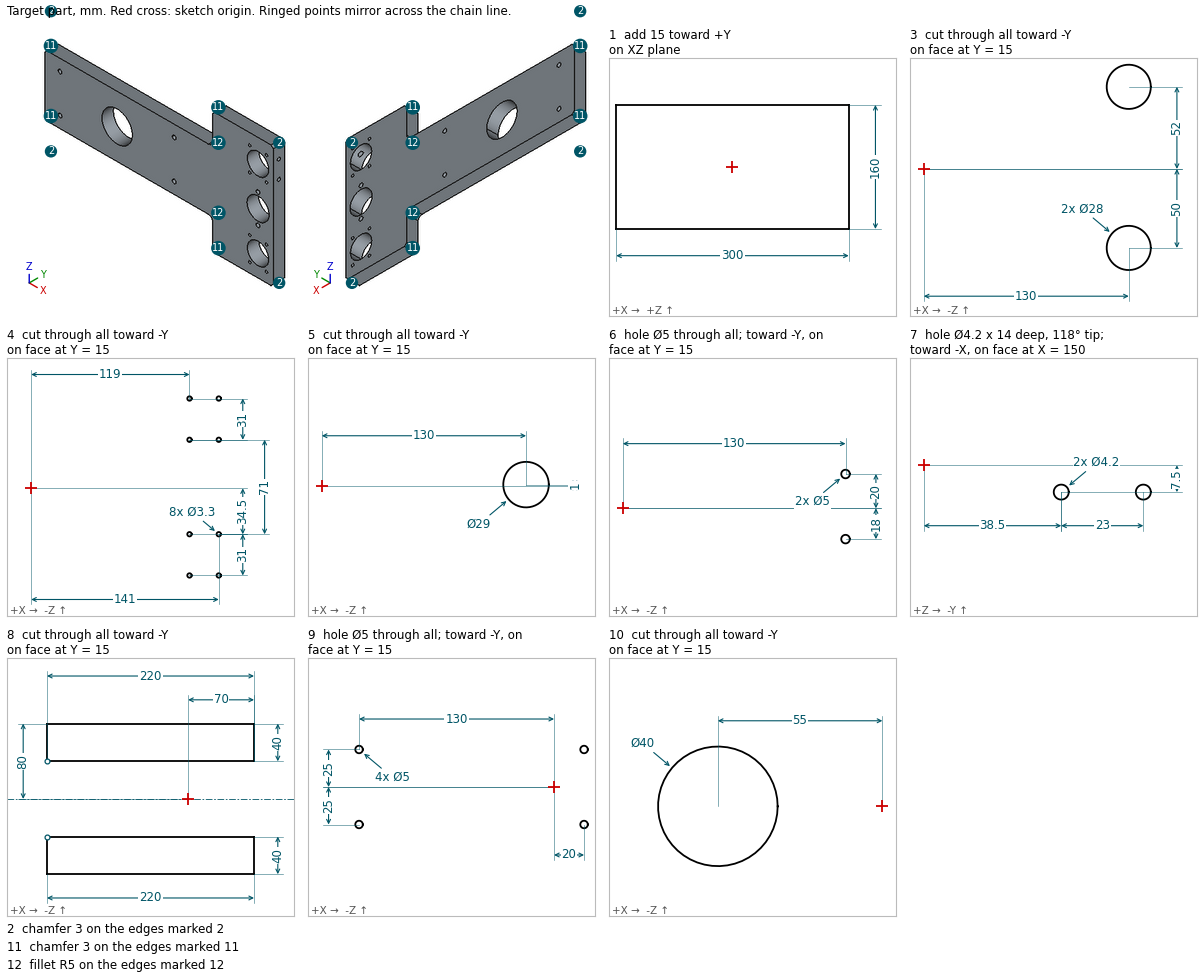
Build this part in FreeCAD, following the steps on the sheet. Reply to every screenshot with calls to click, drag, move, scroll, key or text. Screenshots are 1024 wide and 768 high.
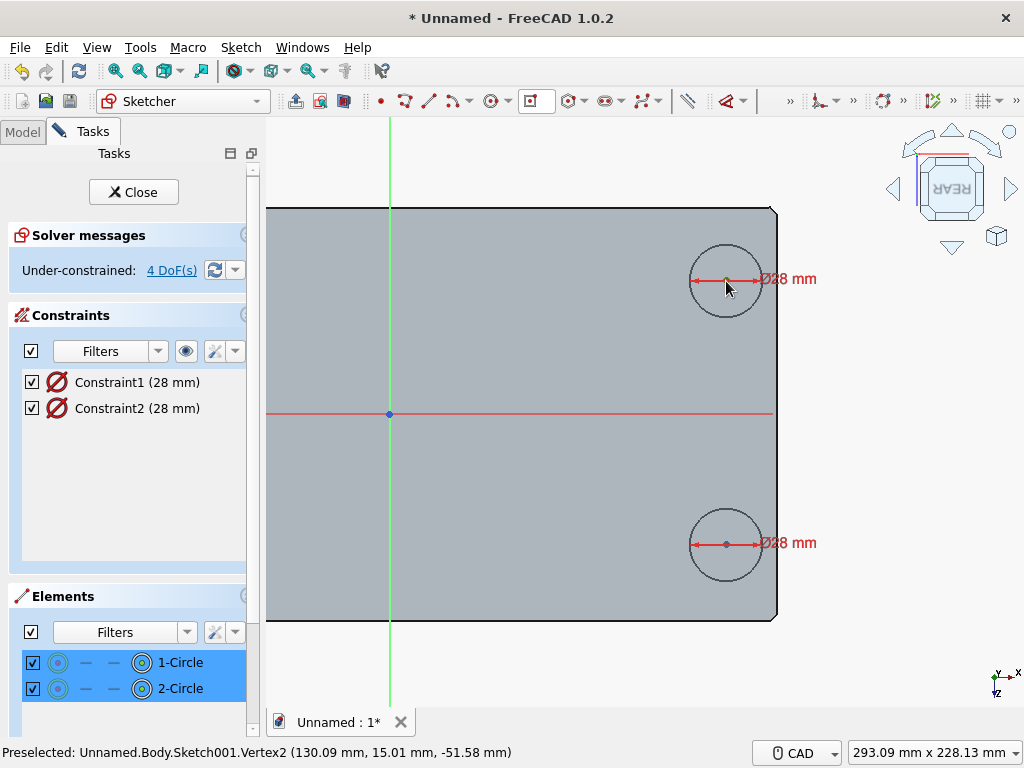
key(v)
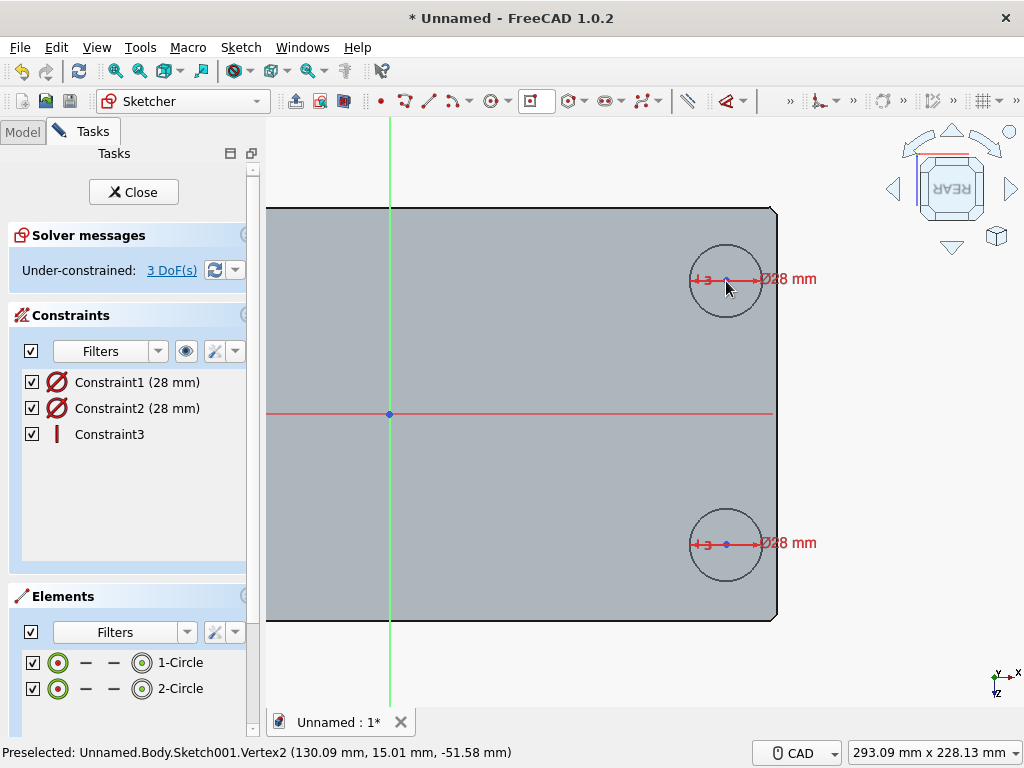
click(726, 102)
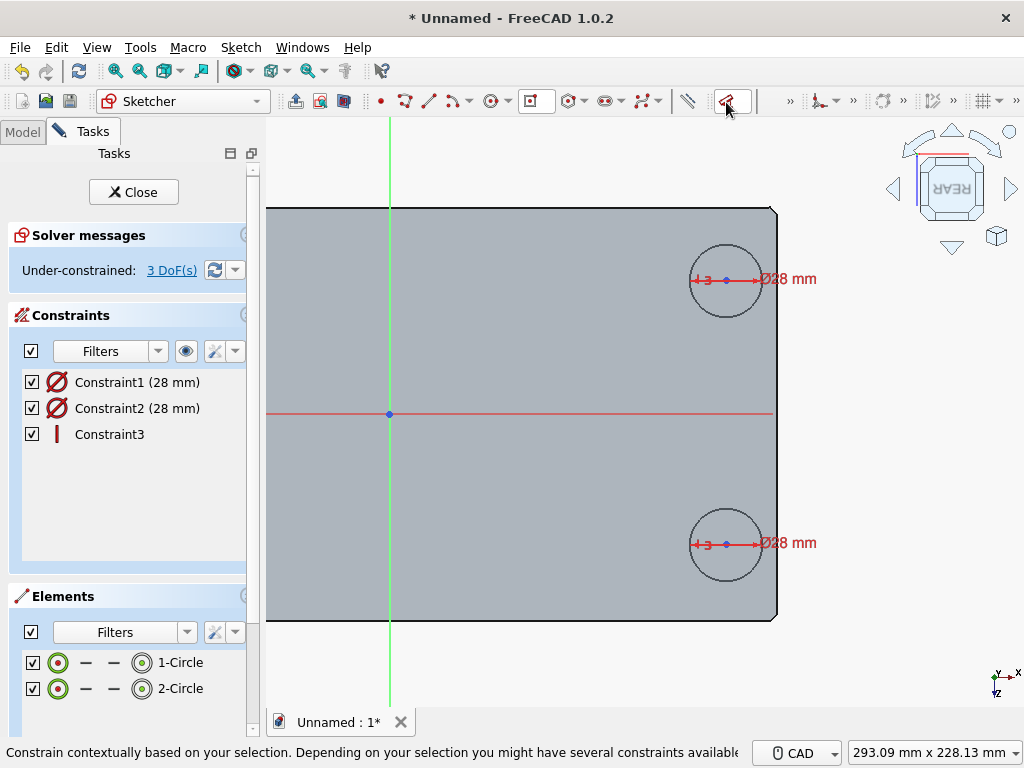
click(726, 545)
click(356, 480)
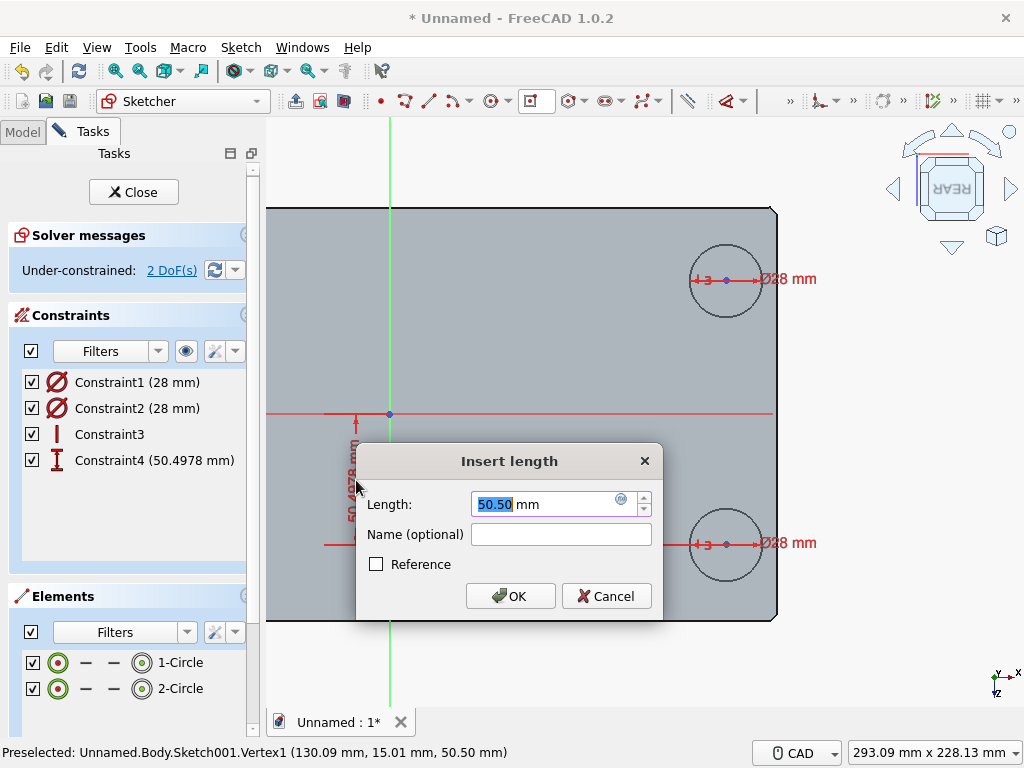
text(50)
key(Return)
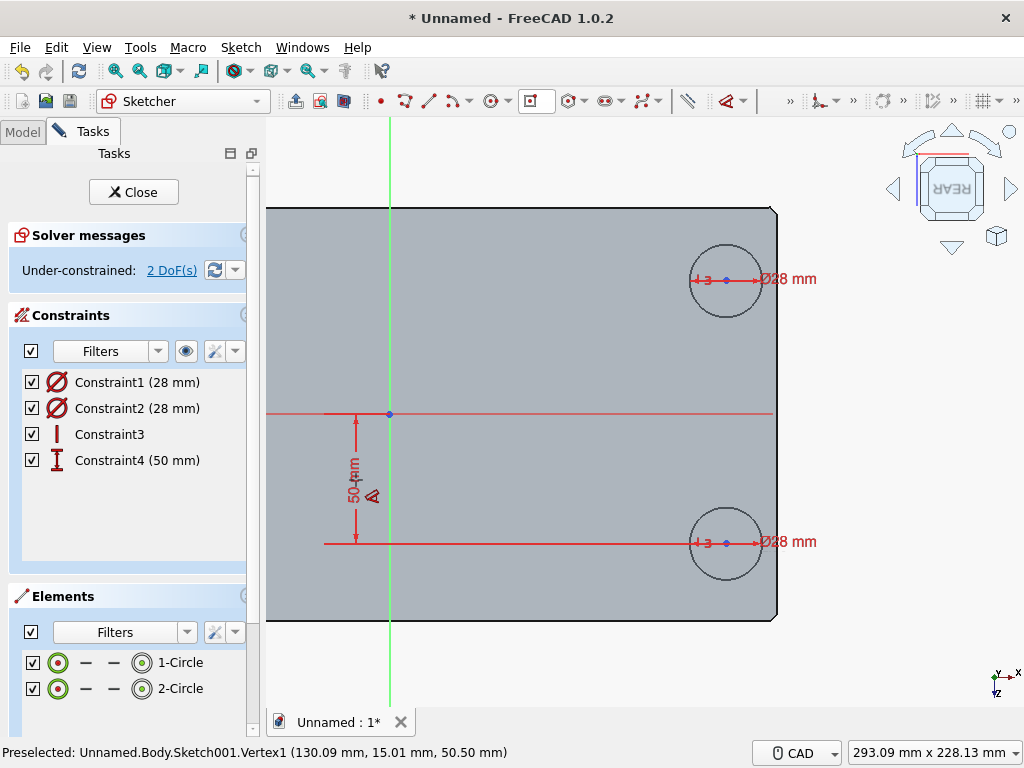
click(726, 281)
click(356, 348)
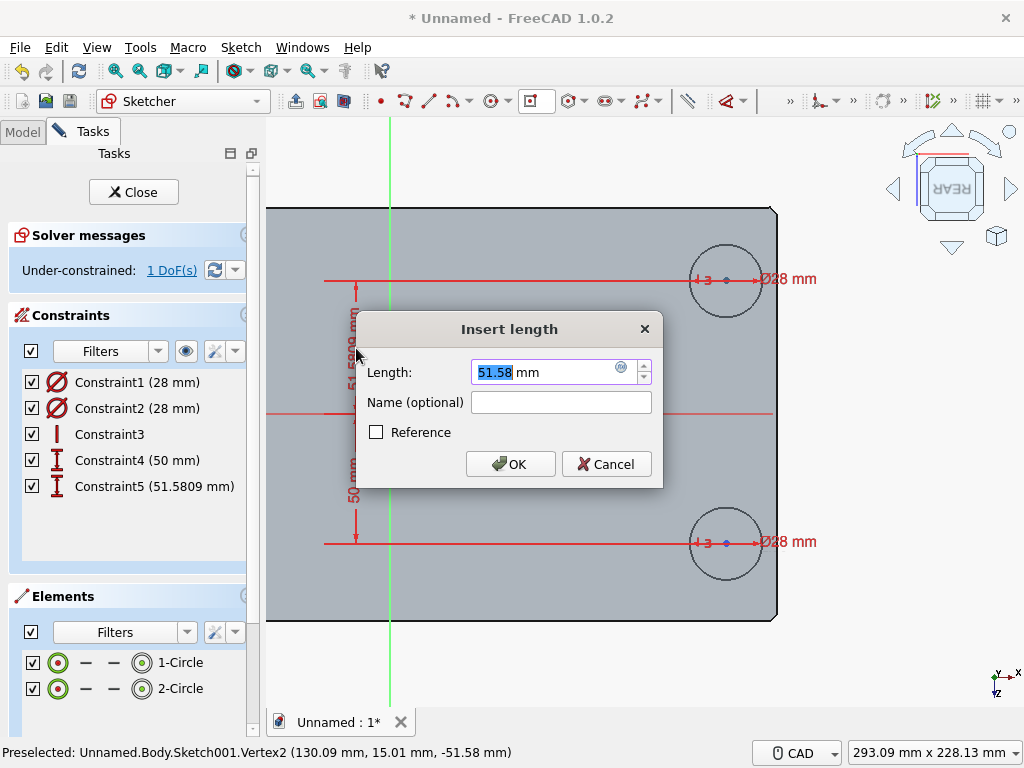
text(52)
key(Return)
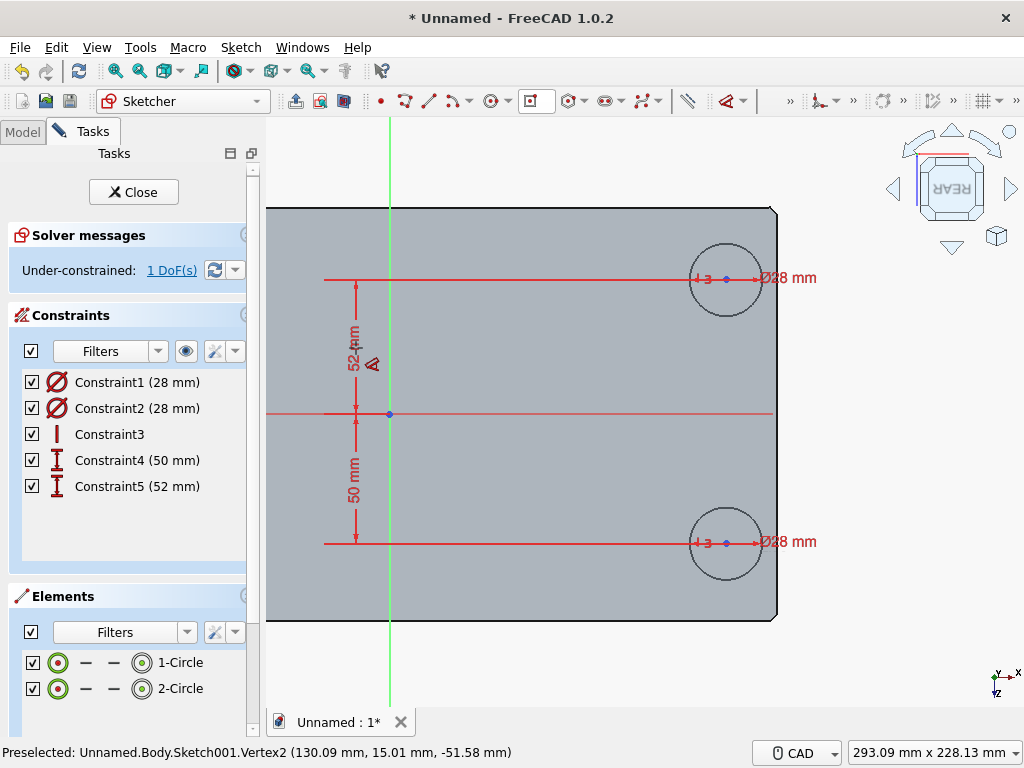
click(726, 544)
click(558, 578)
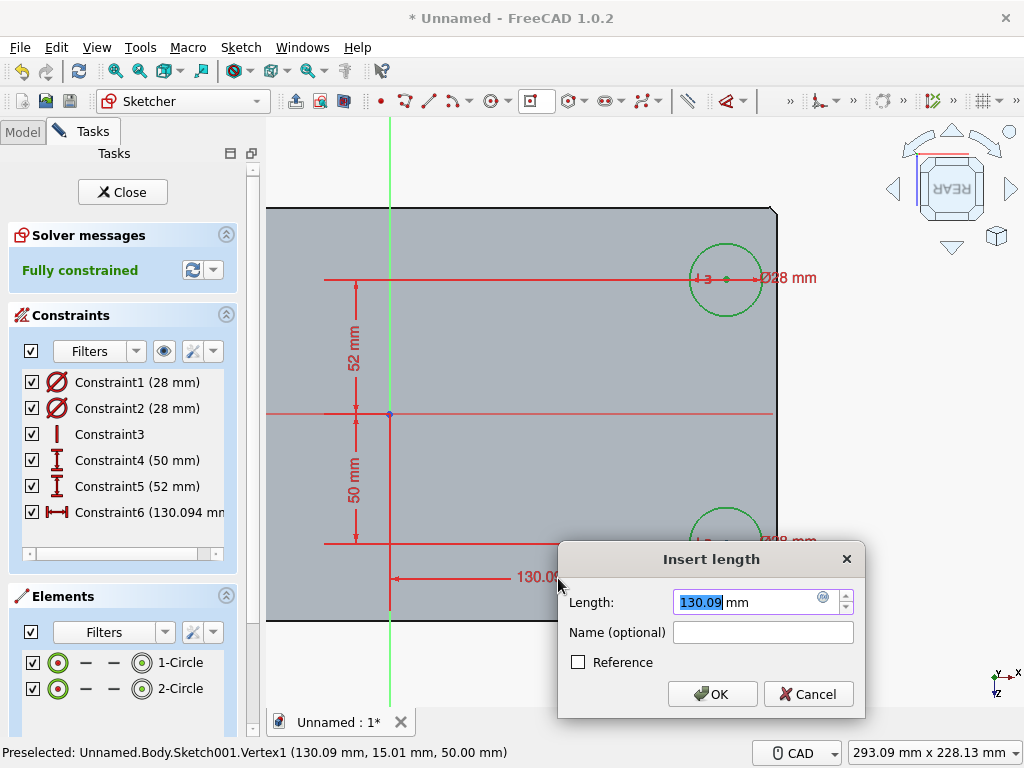
text(130)
key(Return)
key(Escape)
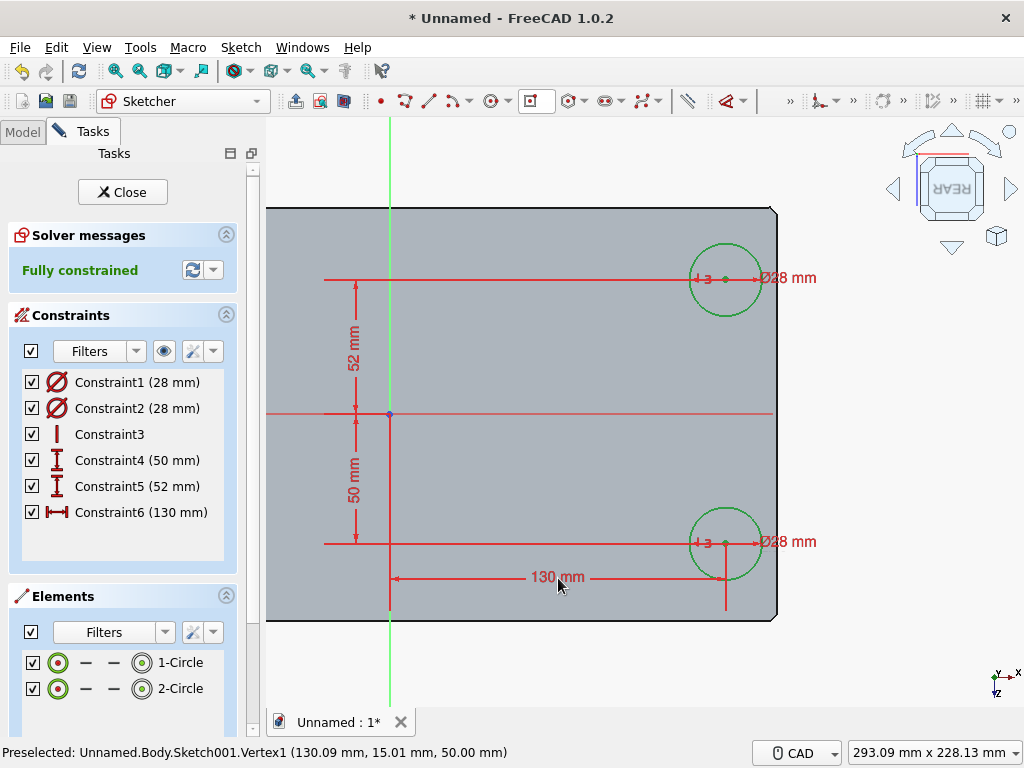
click(123, 192)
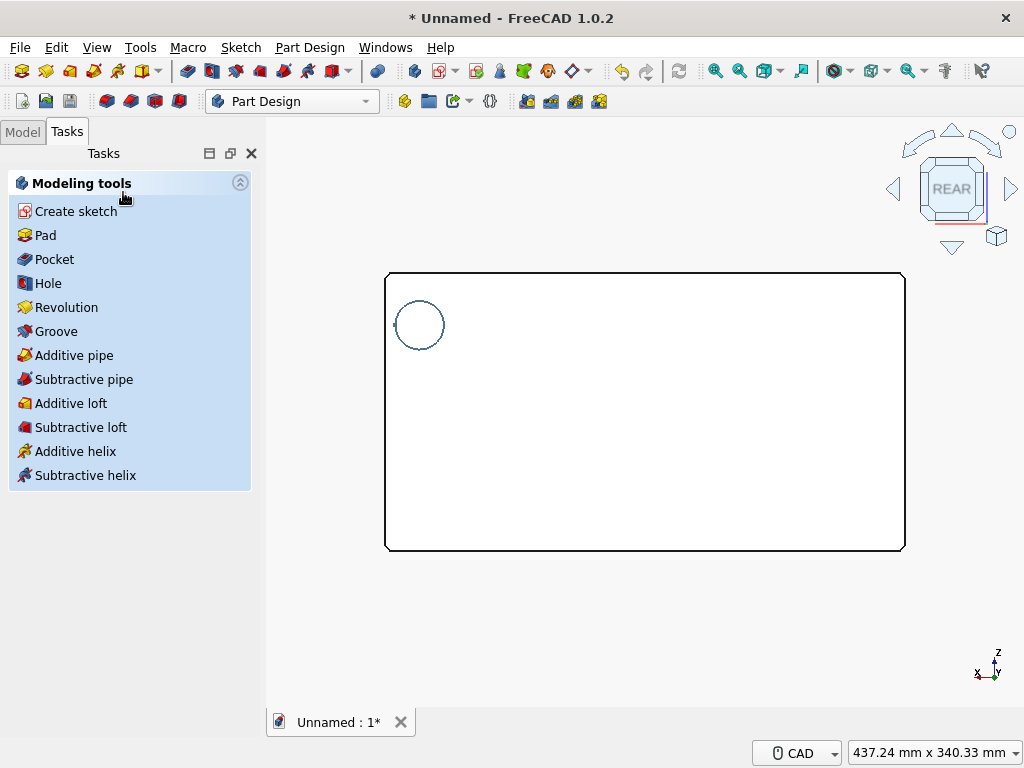
click(188, 72)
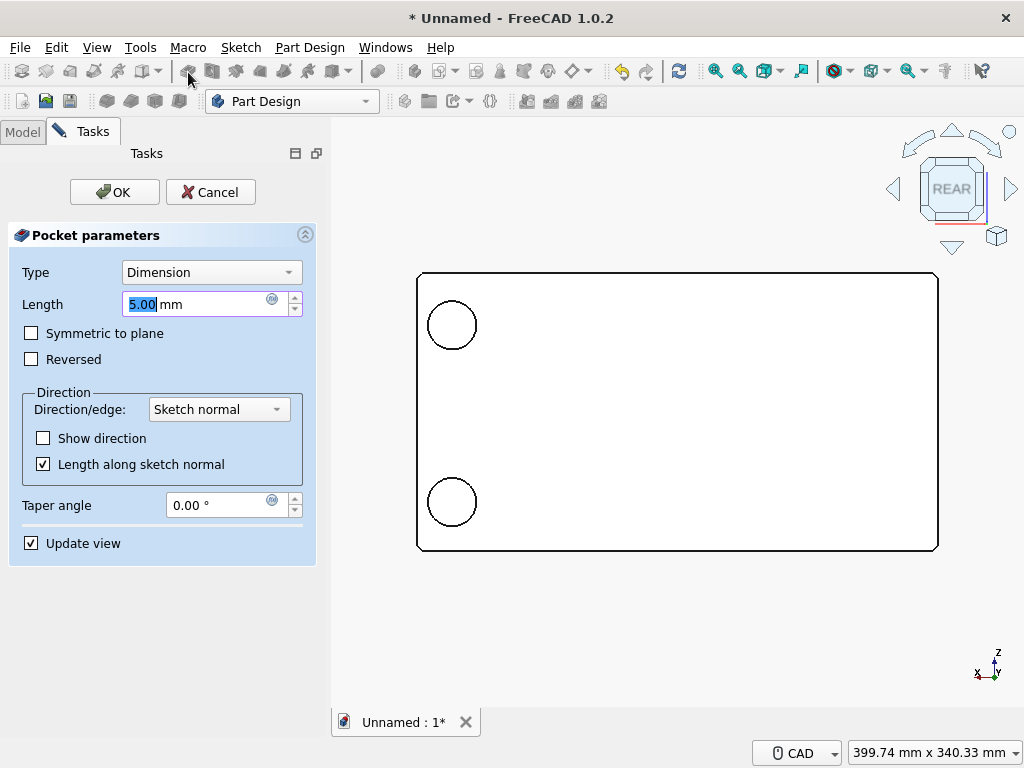
click(212, 272)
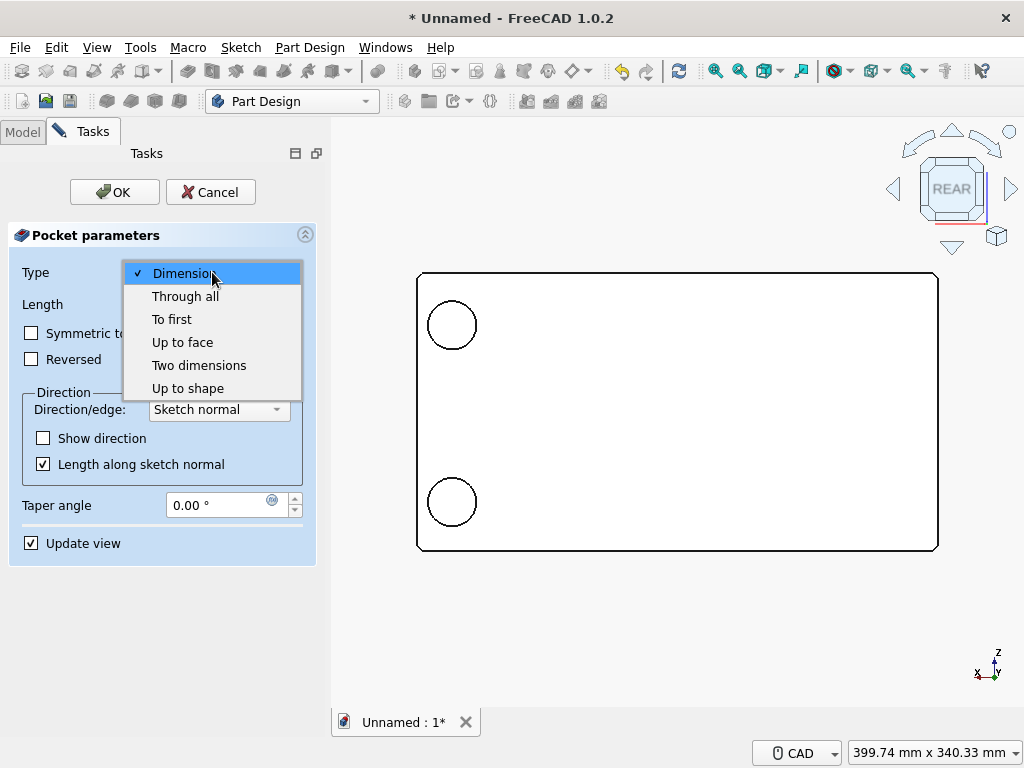
click(212, 296)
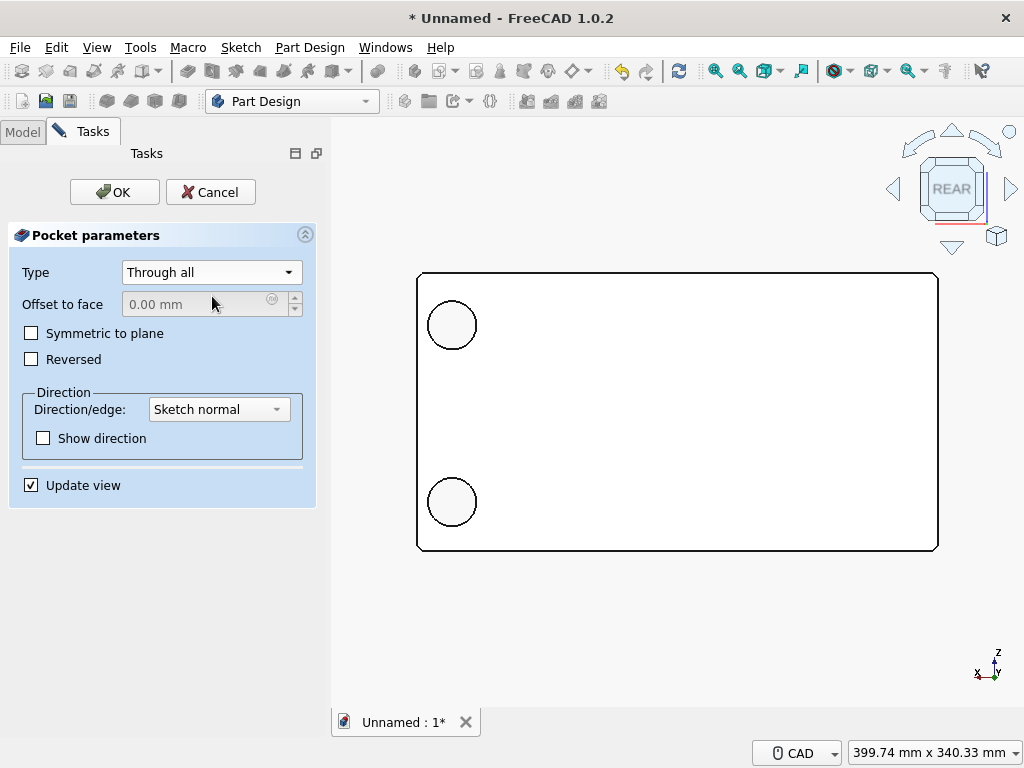
click(115, 192)